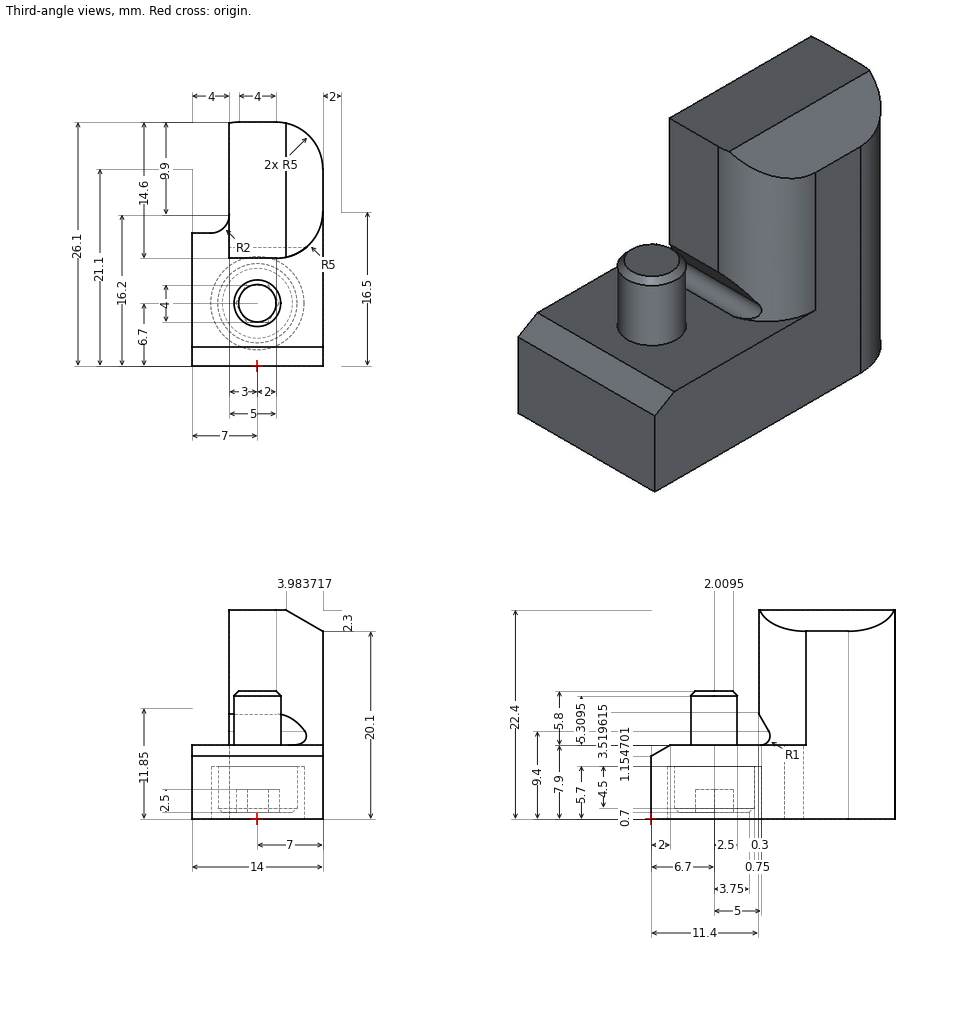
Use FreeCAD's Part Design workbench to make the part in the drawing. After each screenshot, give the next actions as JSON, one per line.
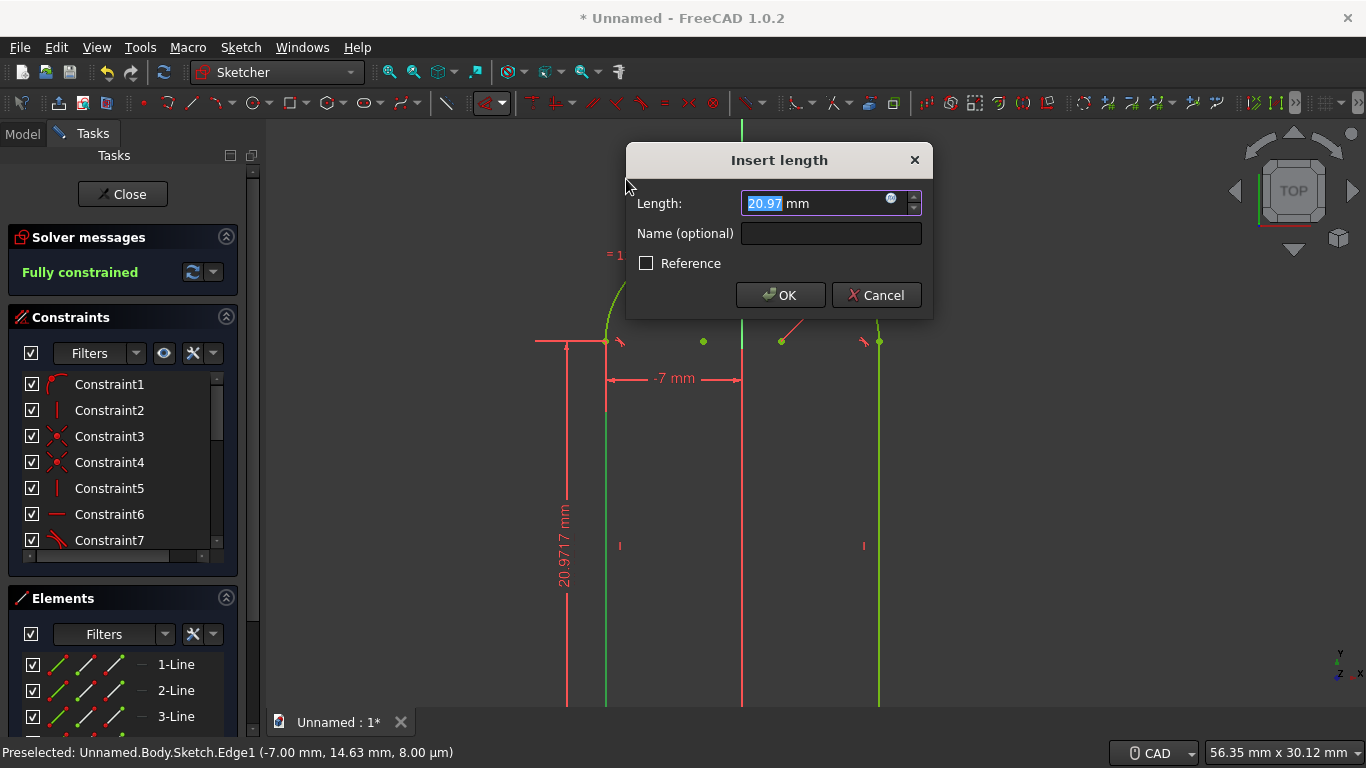
{"action": "type", "text": "21.1"}
{"action": "key", "text": "Return"}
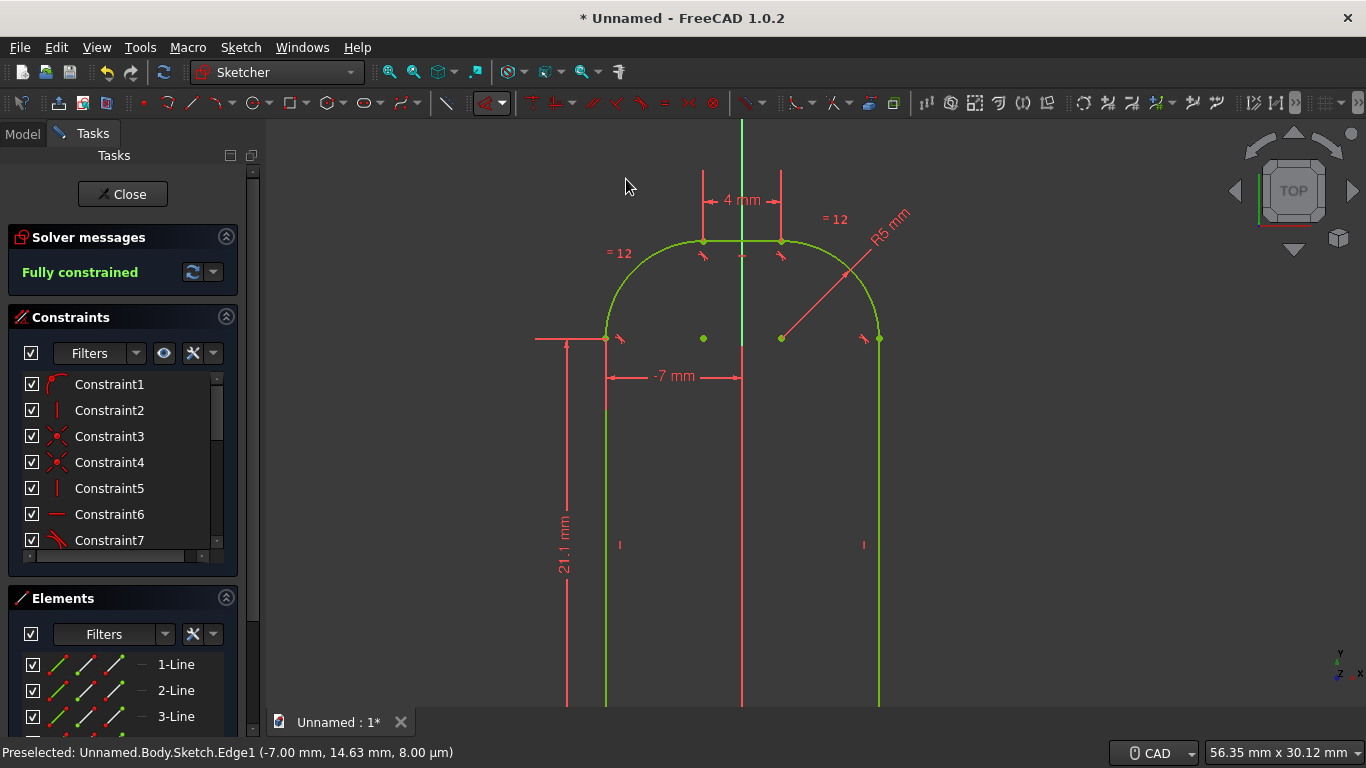
{"action": "left_click", "coordinate": [123, 194]}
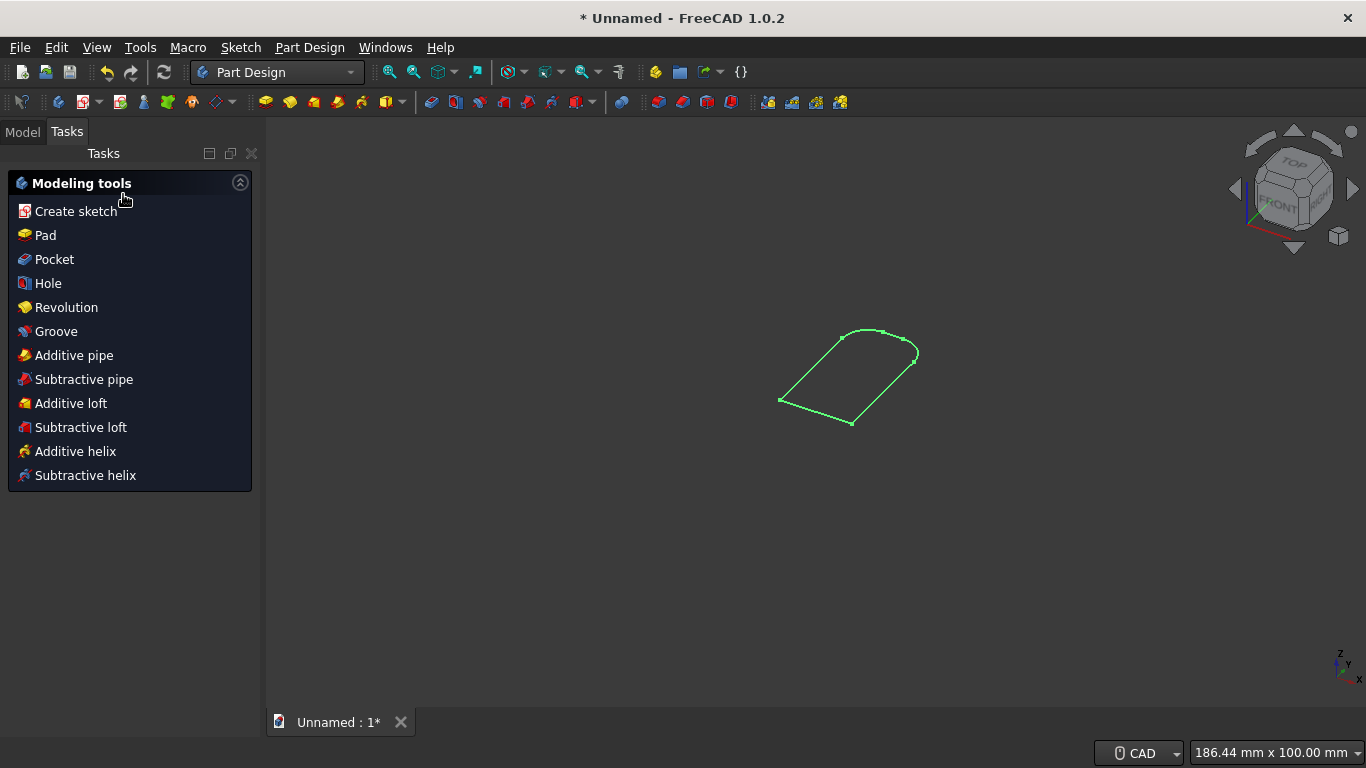
{"action": "left_click", "coordinate": [266, 102]}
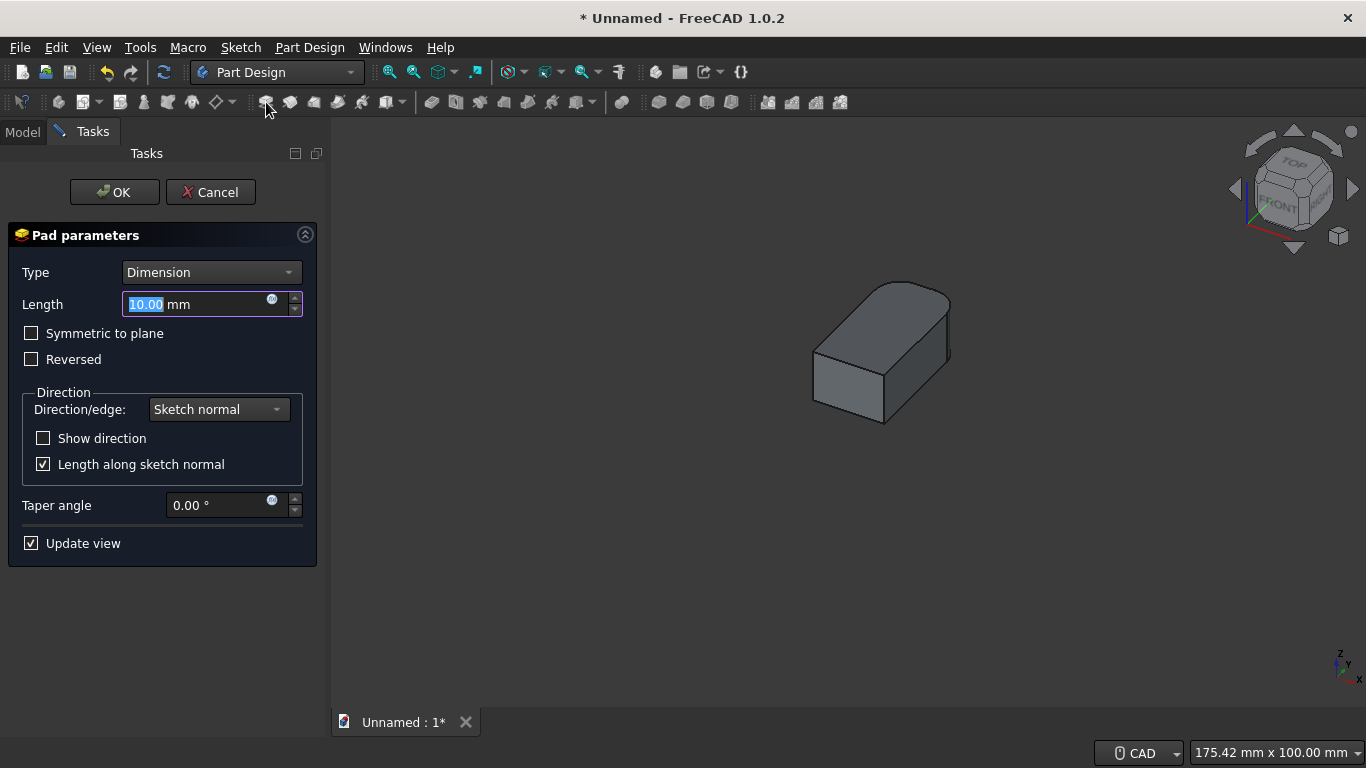
{"action": "type", "text": "22.4"}
{"action": "key", "text": "Tab"}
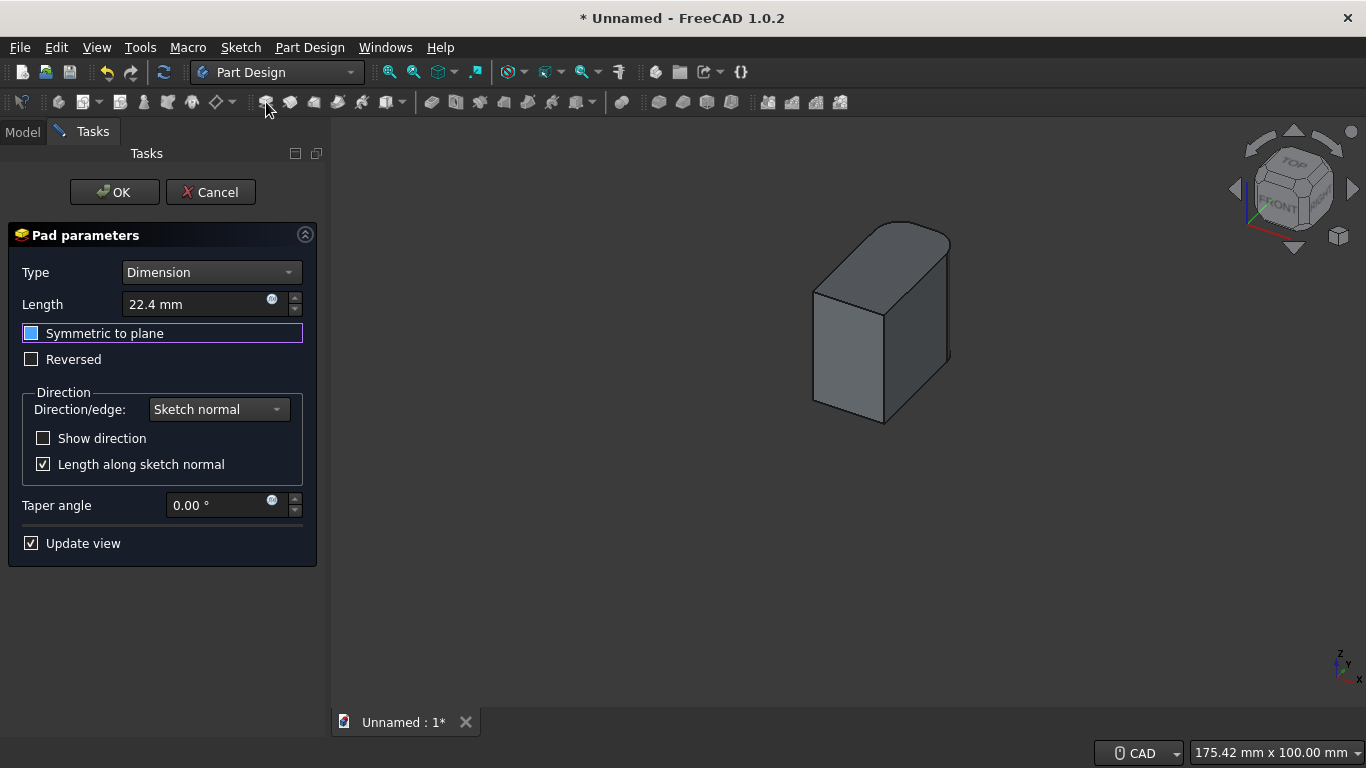
{"action": "left_click", "coordinate": [115, 192]}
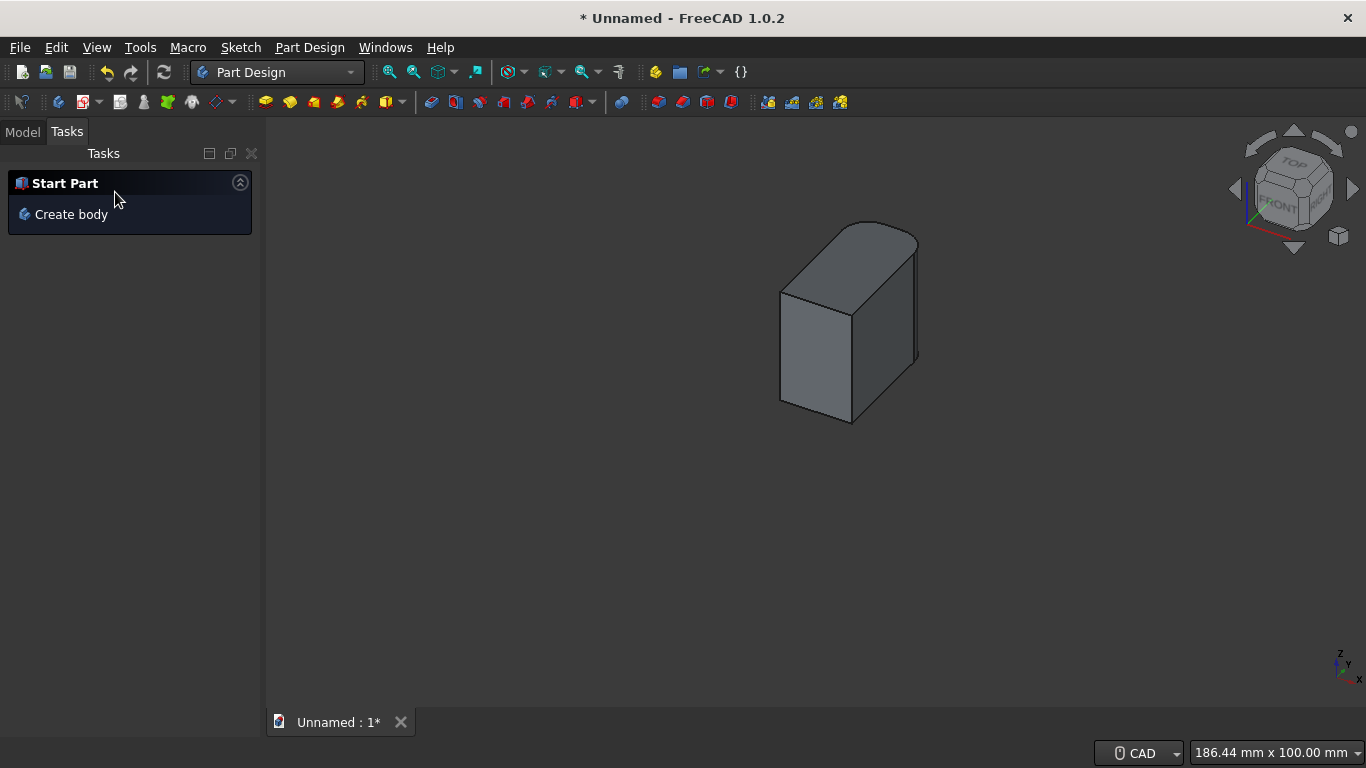
{"action": "left_click", "coordinate": [390, 72]}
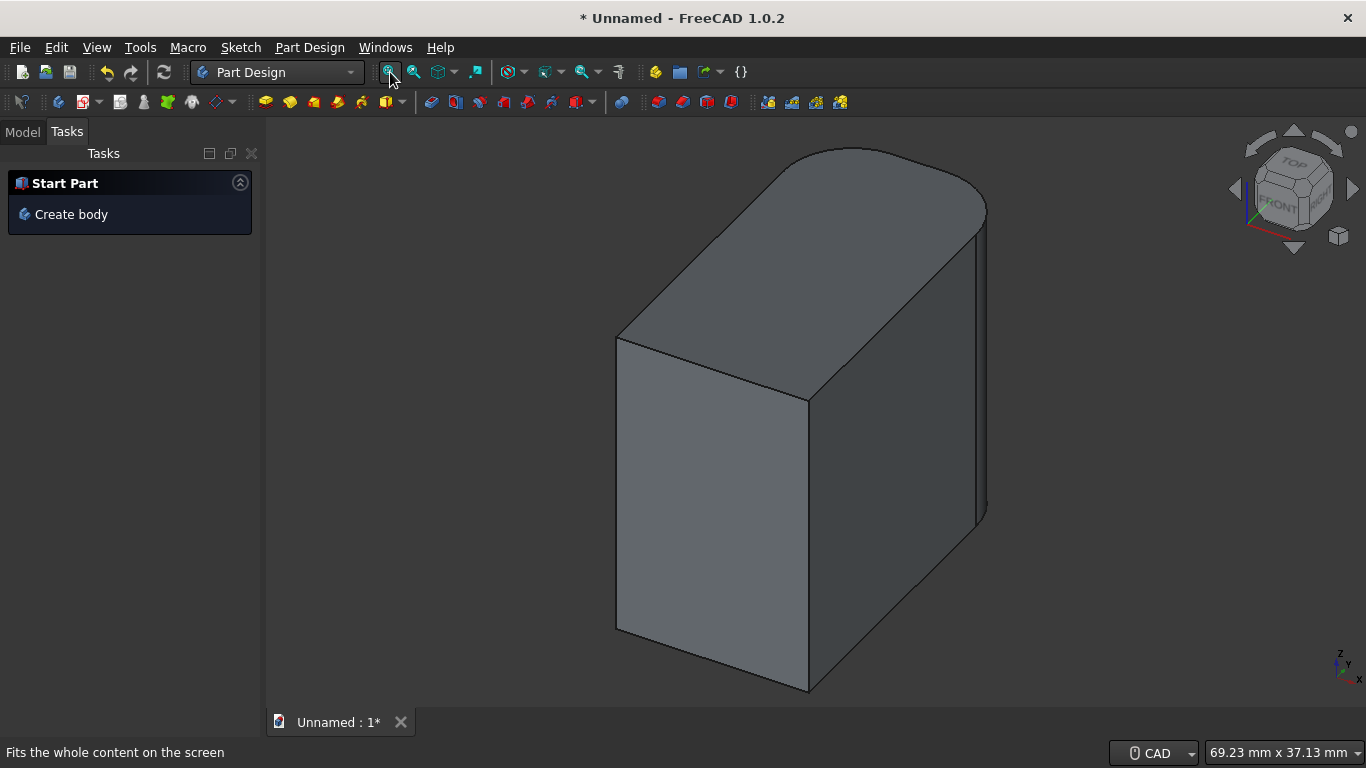
{"action": "left_click", "coordinate": [84, 102]}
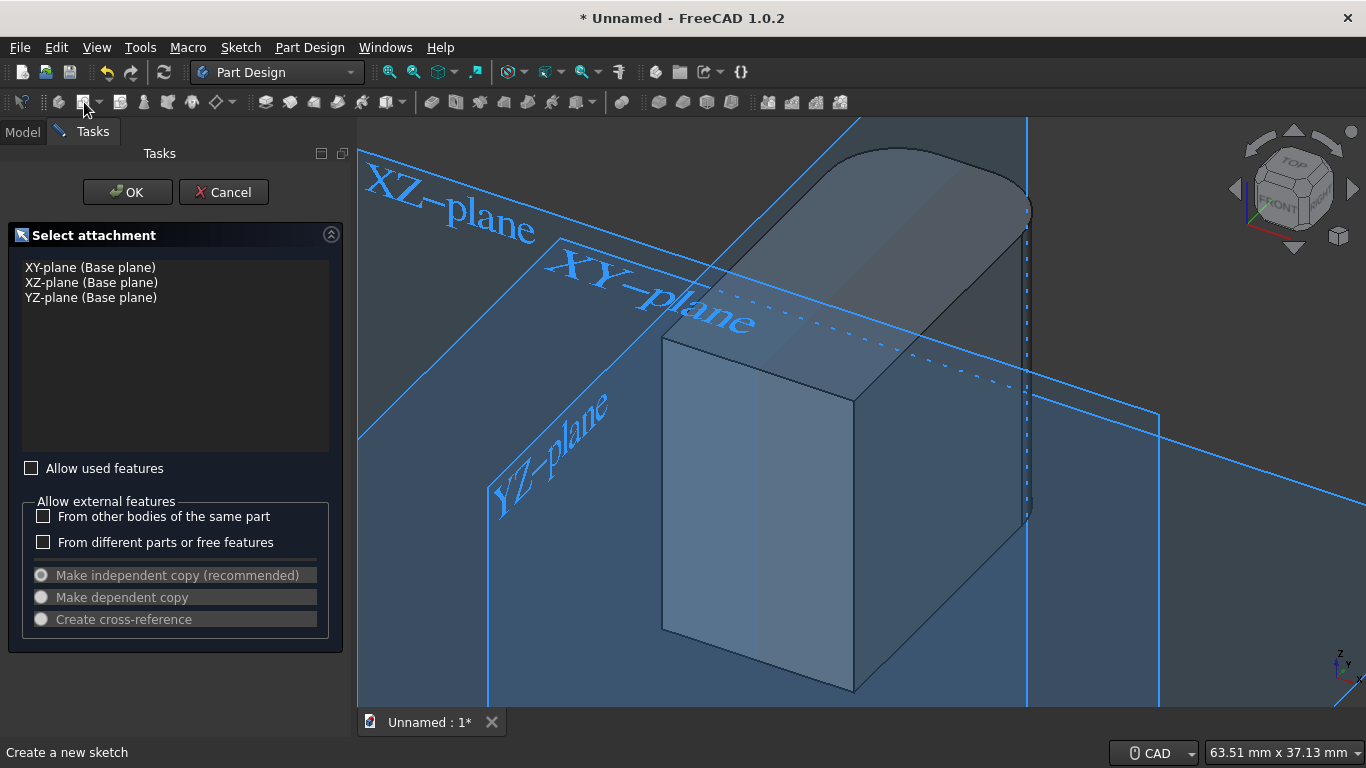
{"action": "left_click", "coordinate": [82, 298]}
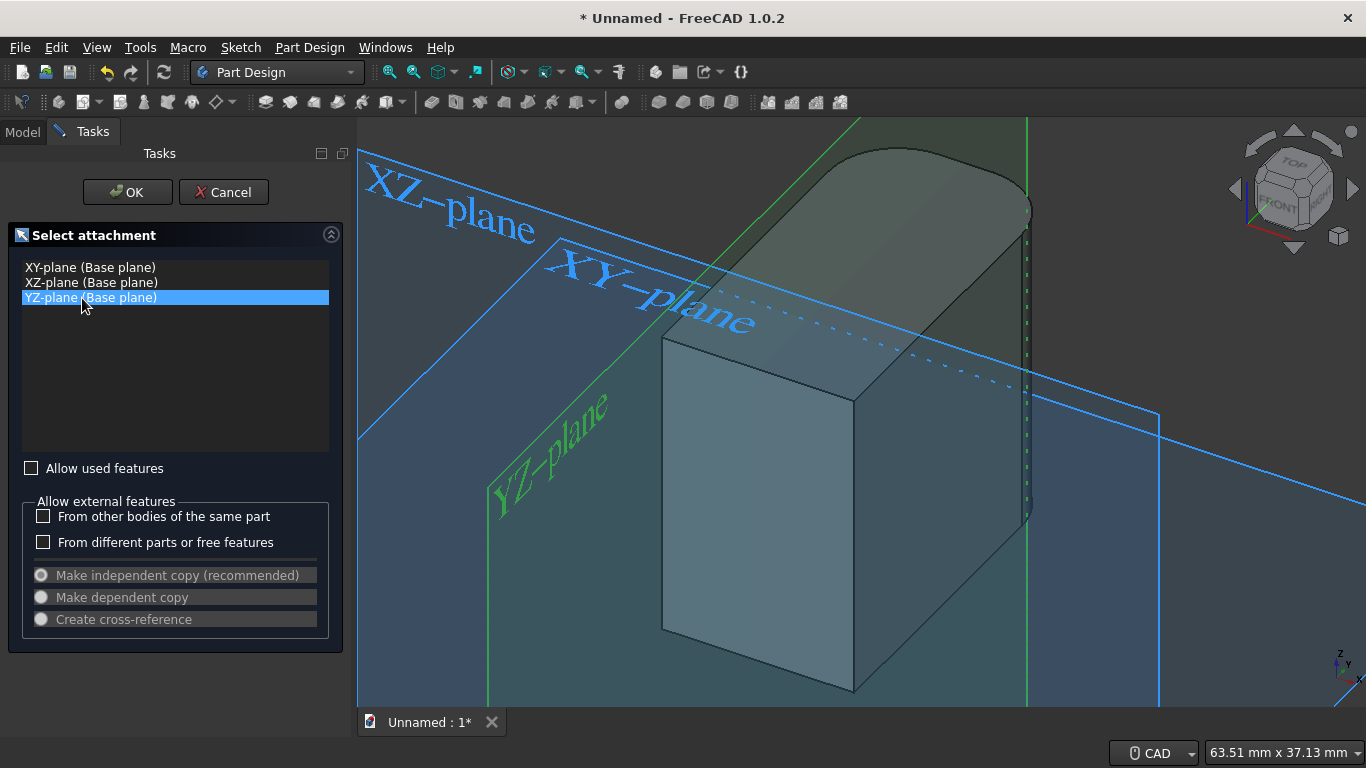
{"action": "left_click", "coordinate": [128, 192]}